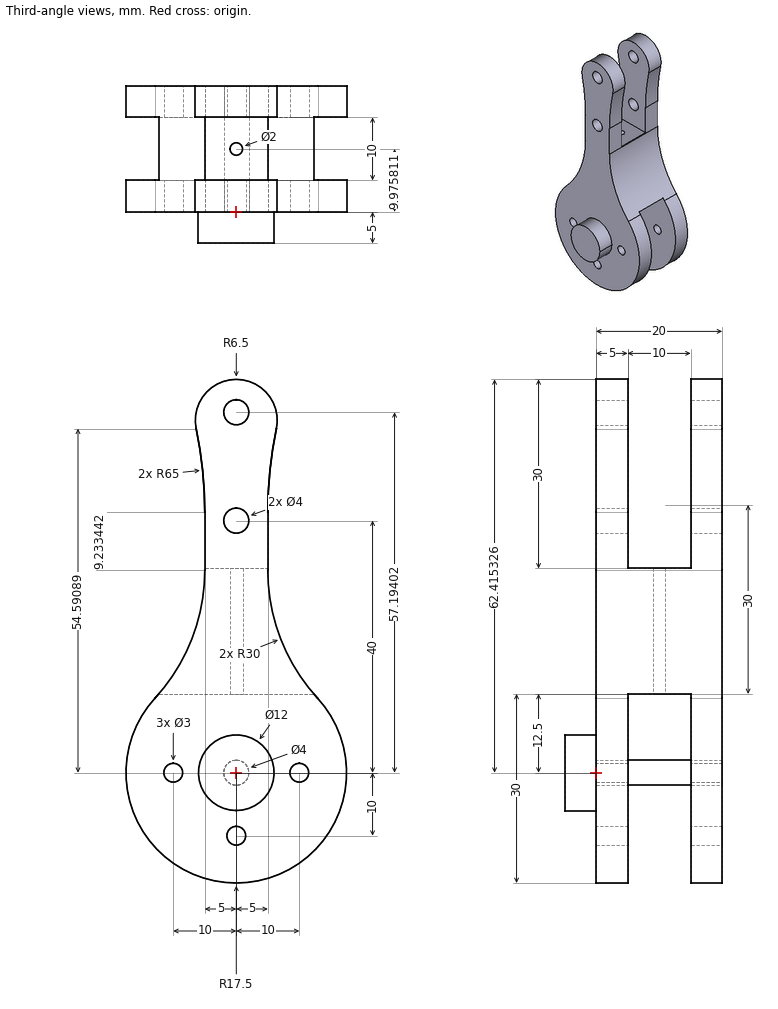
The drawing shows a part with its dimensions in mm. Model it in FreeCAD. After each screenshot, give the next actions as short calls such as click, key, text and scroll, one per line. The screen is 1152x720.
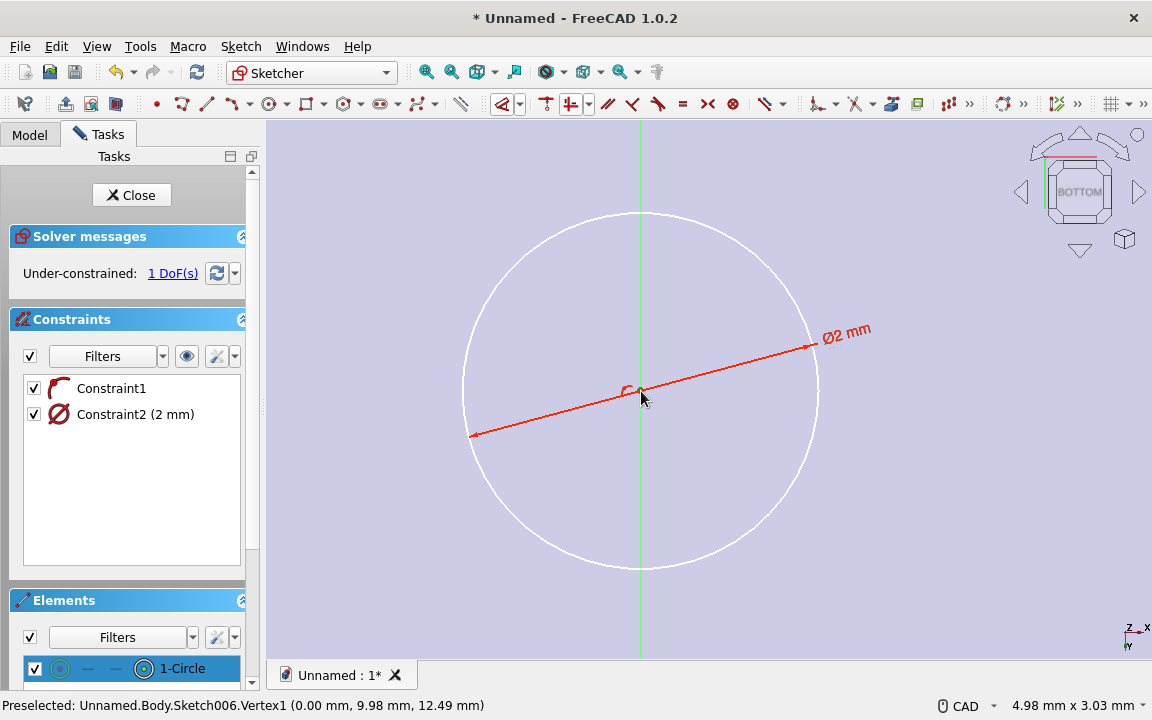
key(i)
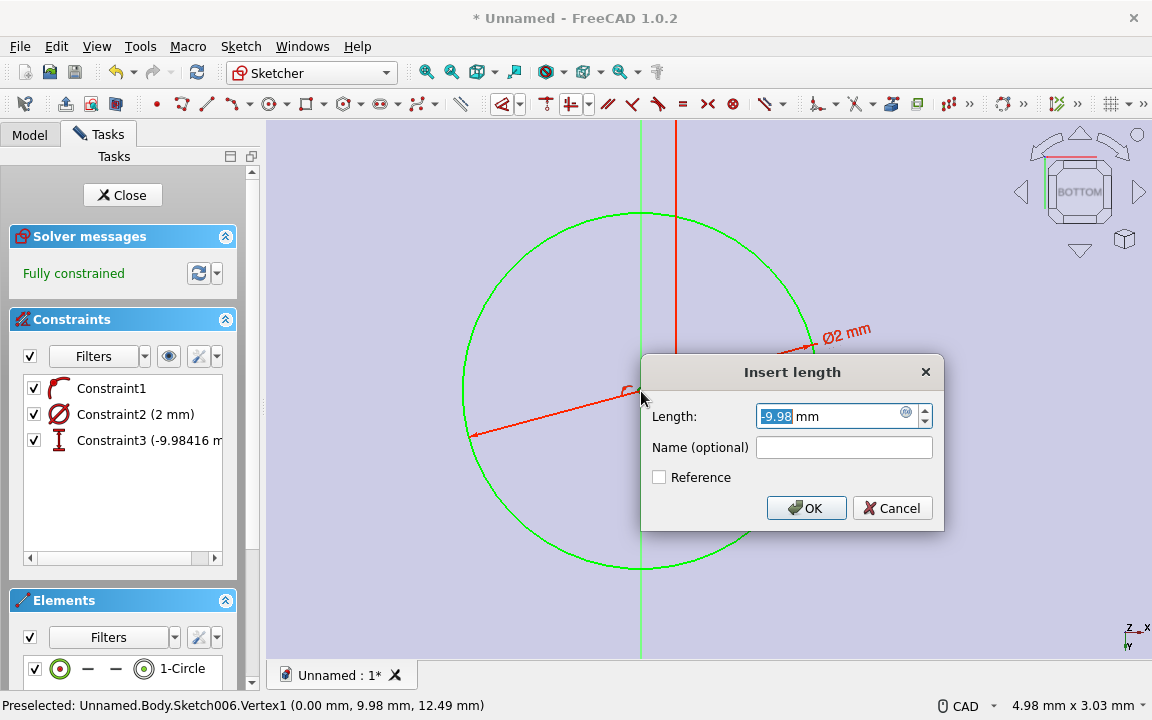
text(-9.975811)
key(Return)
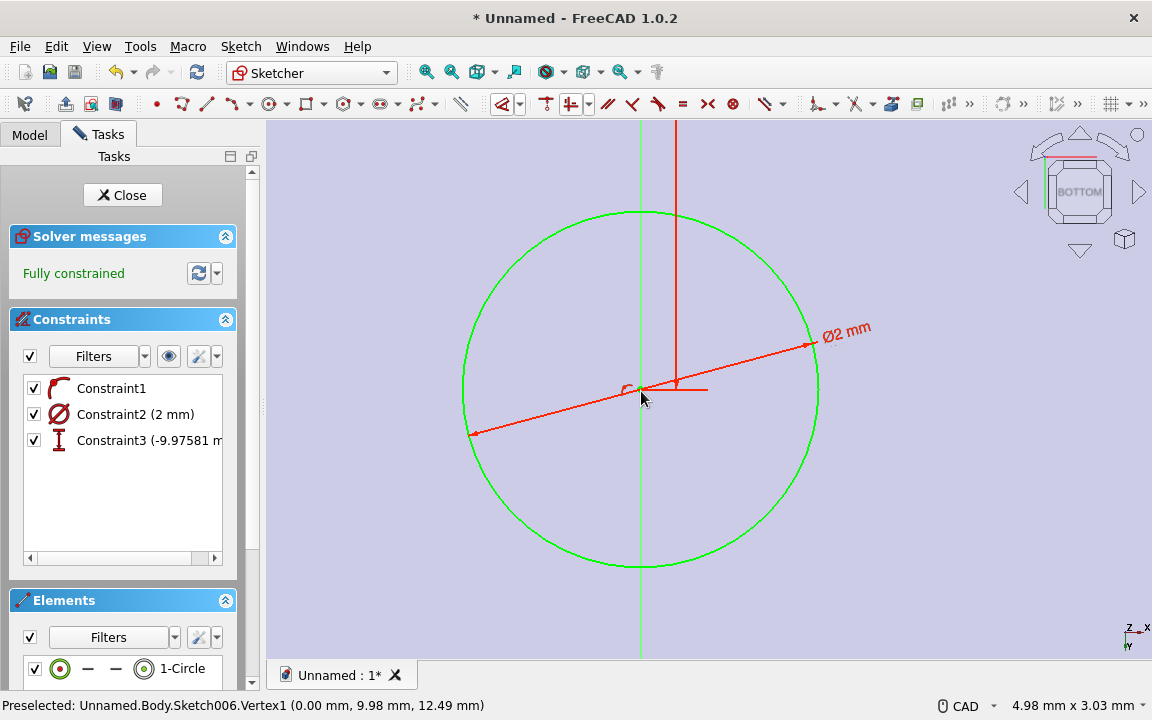
click(123, 195)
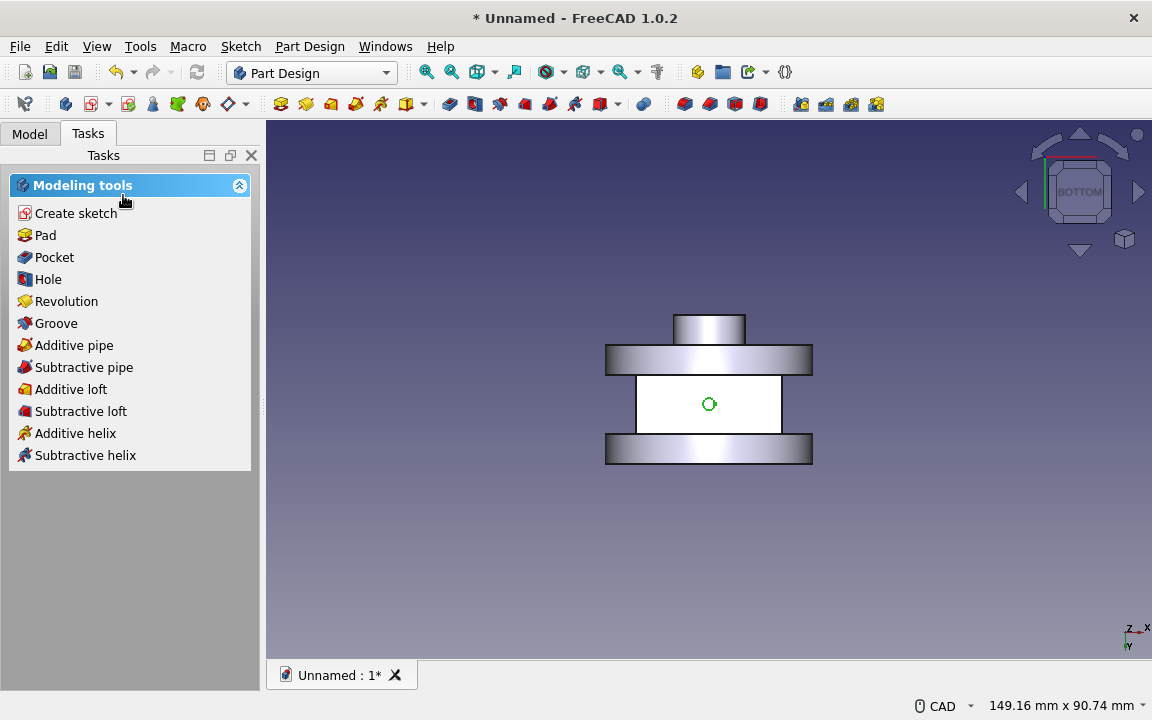
click(450, 104)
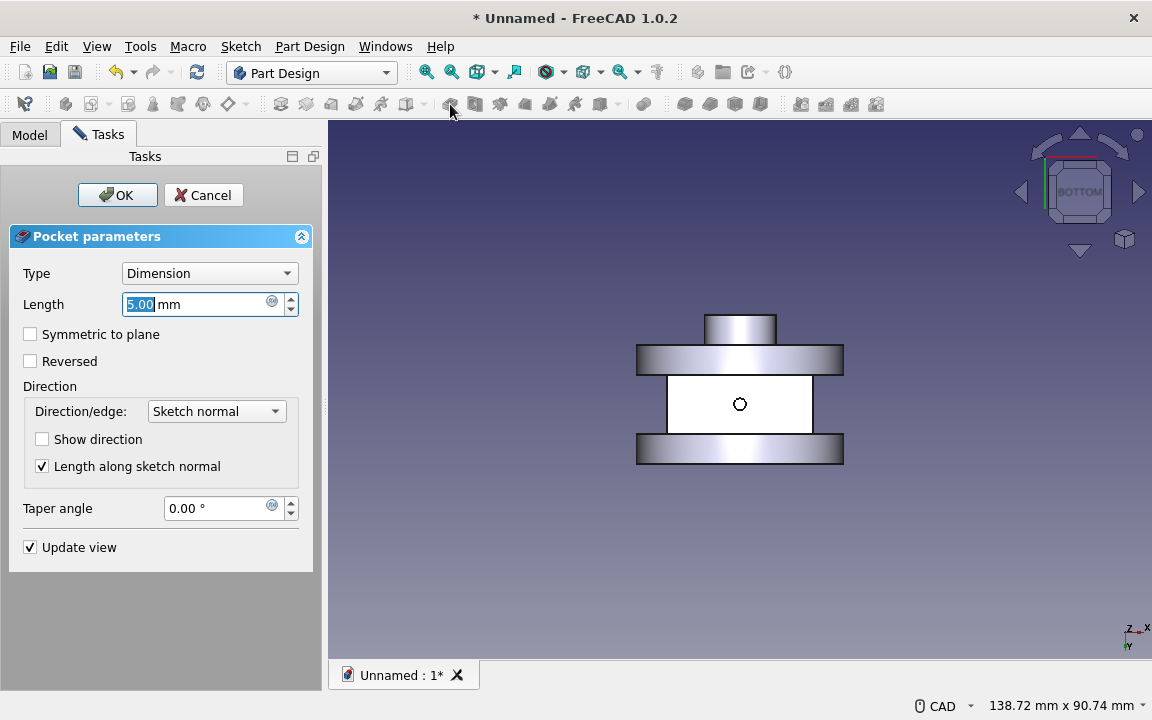
text(30)
key(Tab)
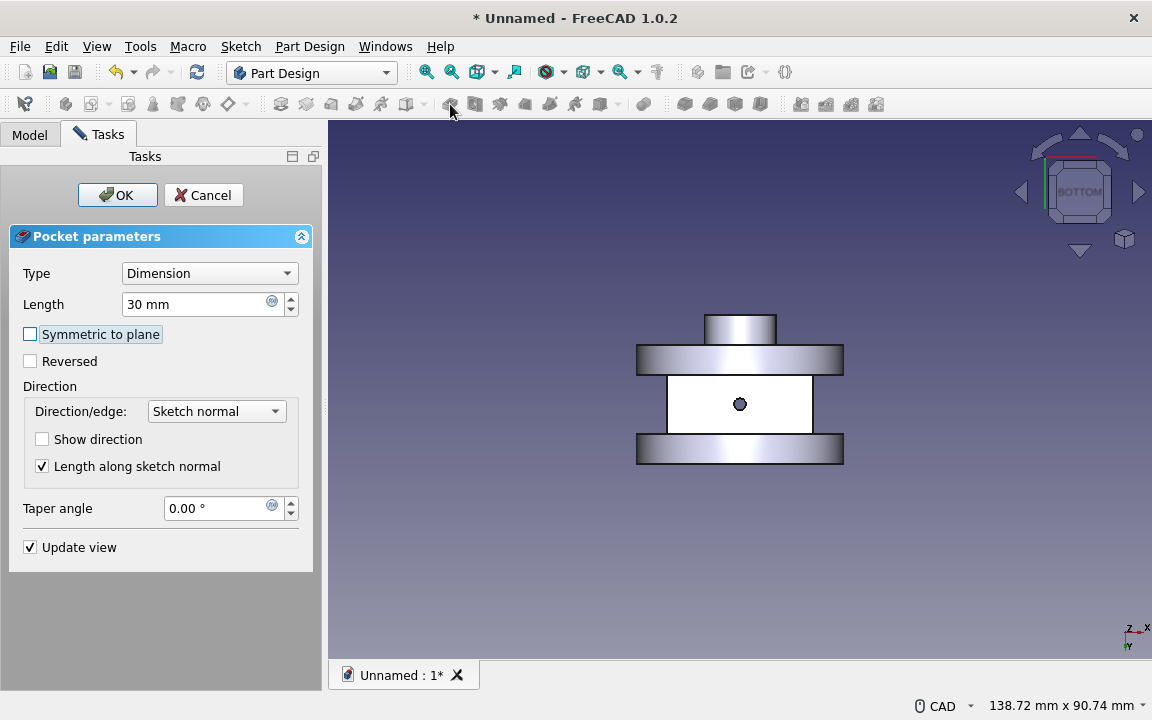
click(118, 195)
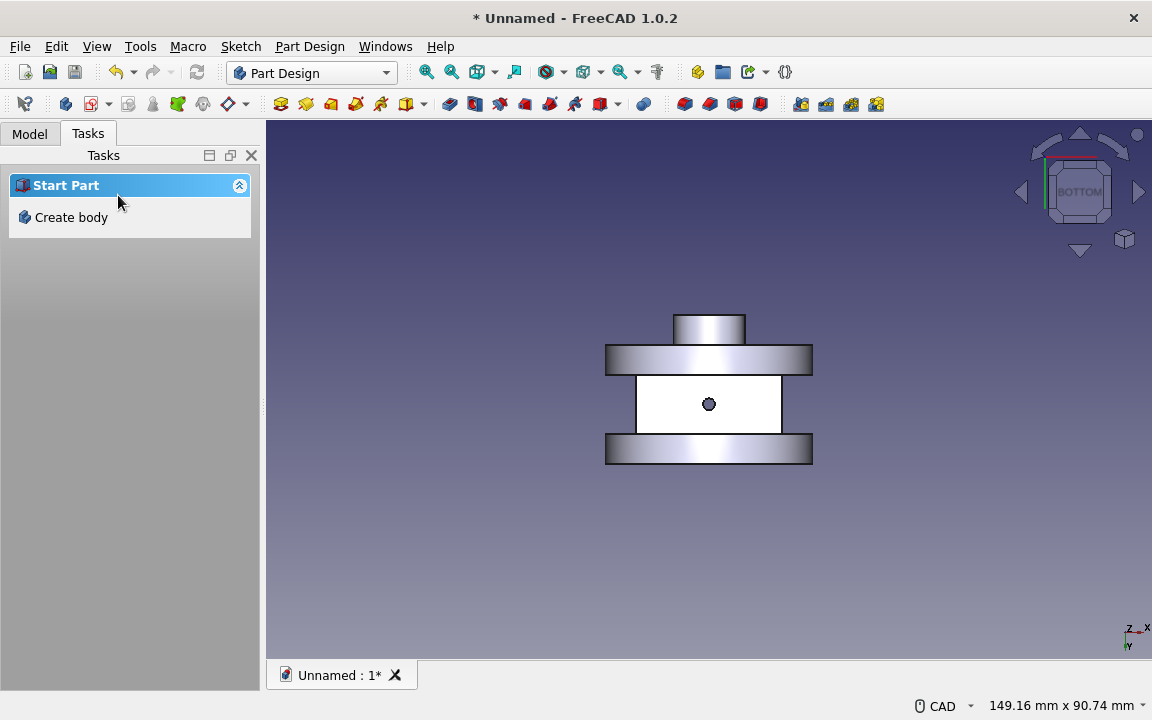
click(427, 72)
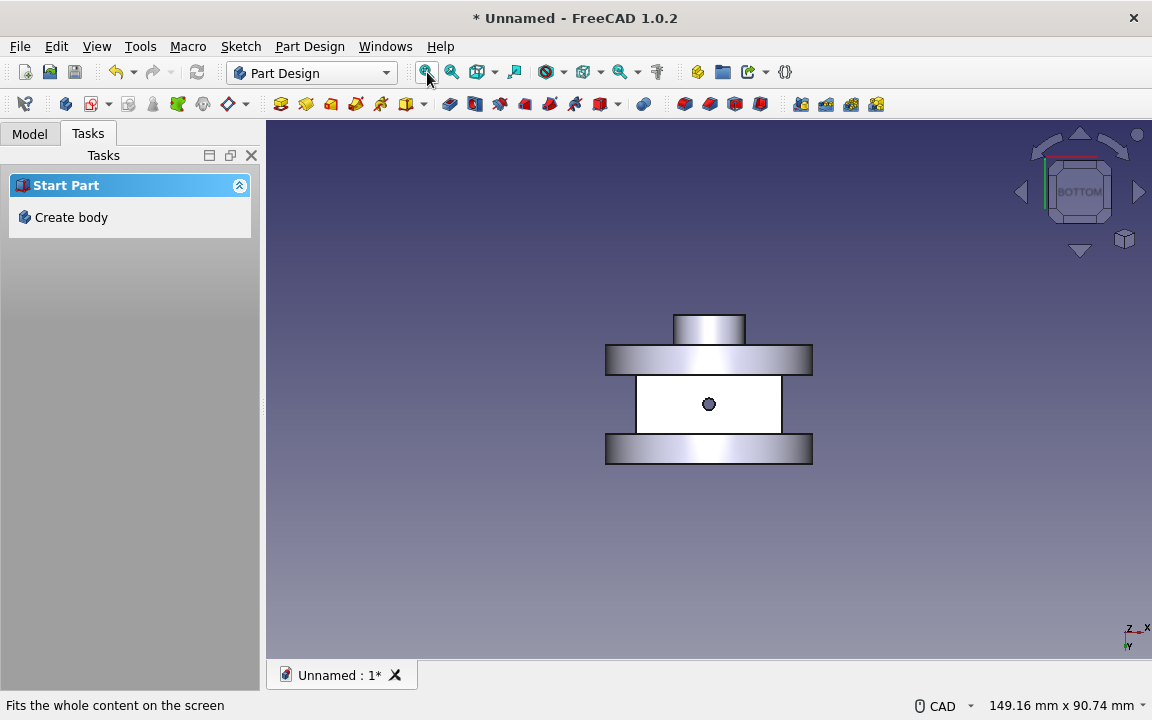
click(66, 104)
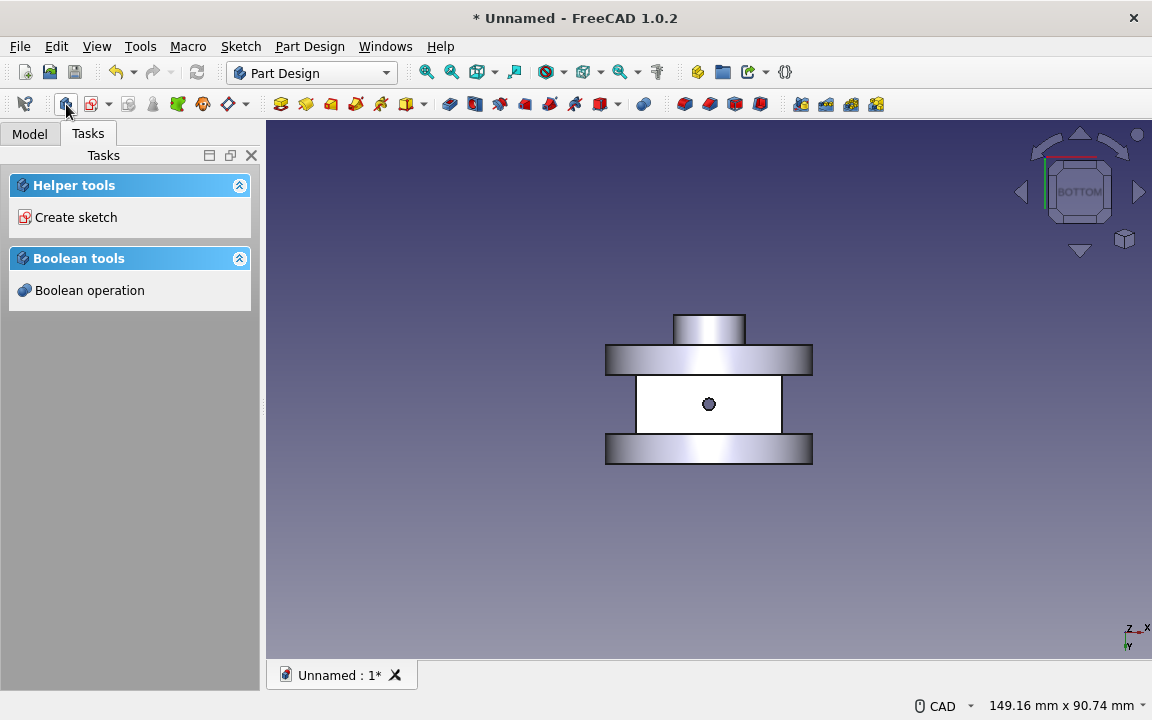
click(30, 134)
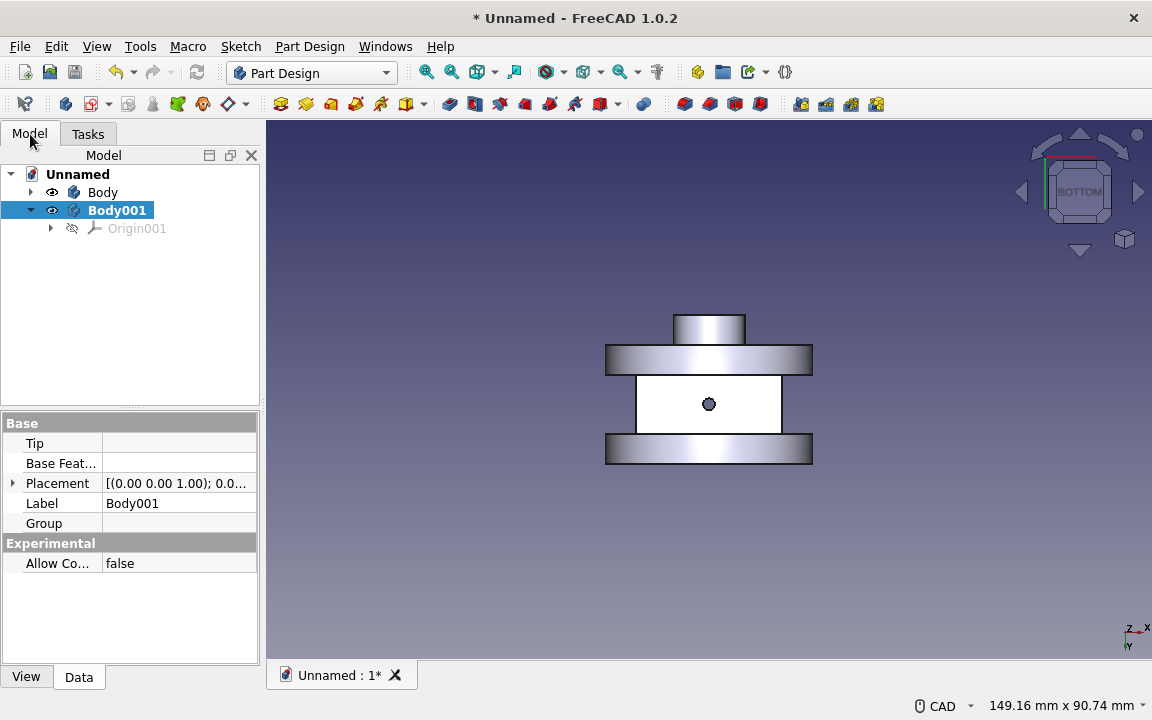
click(51, 228)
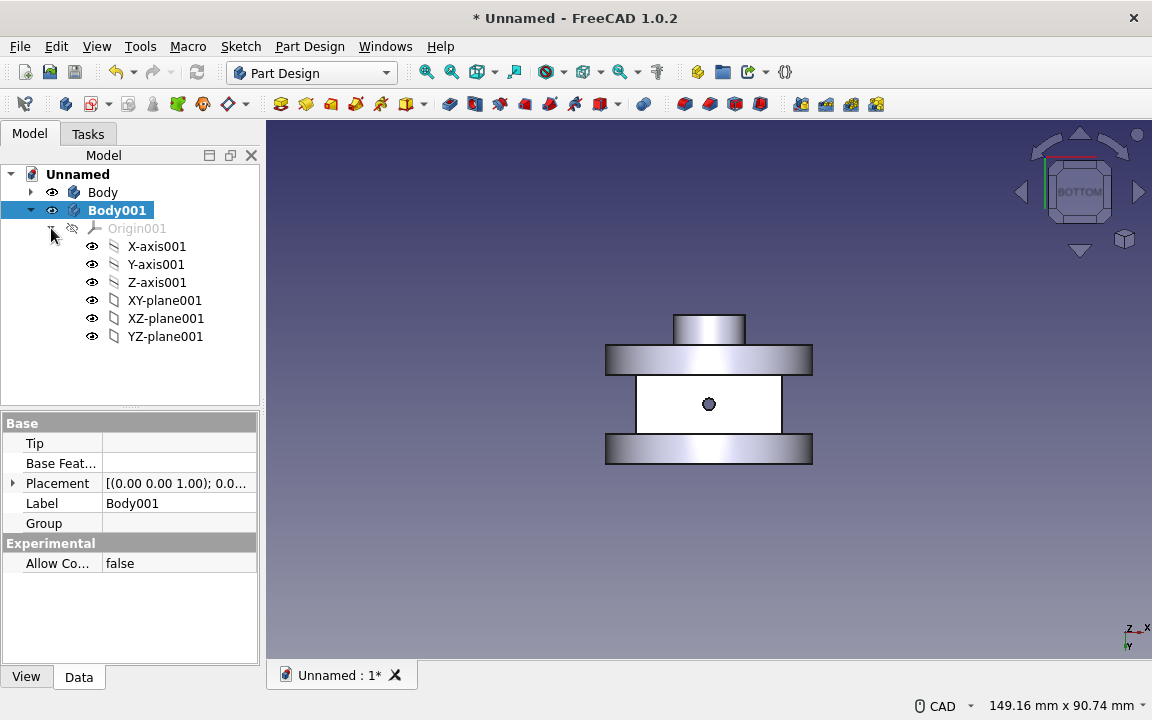
click(137, 318)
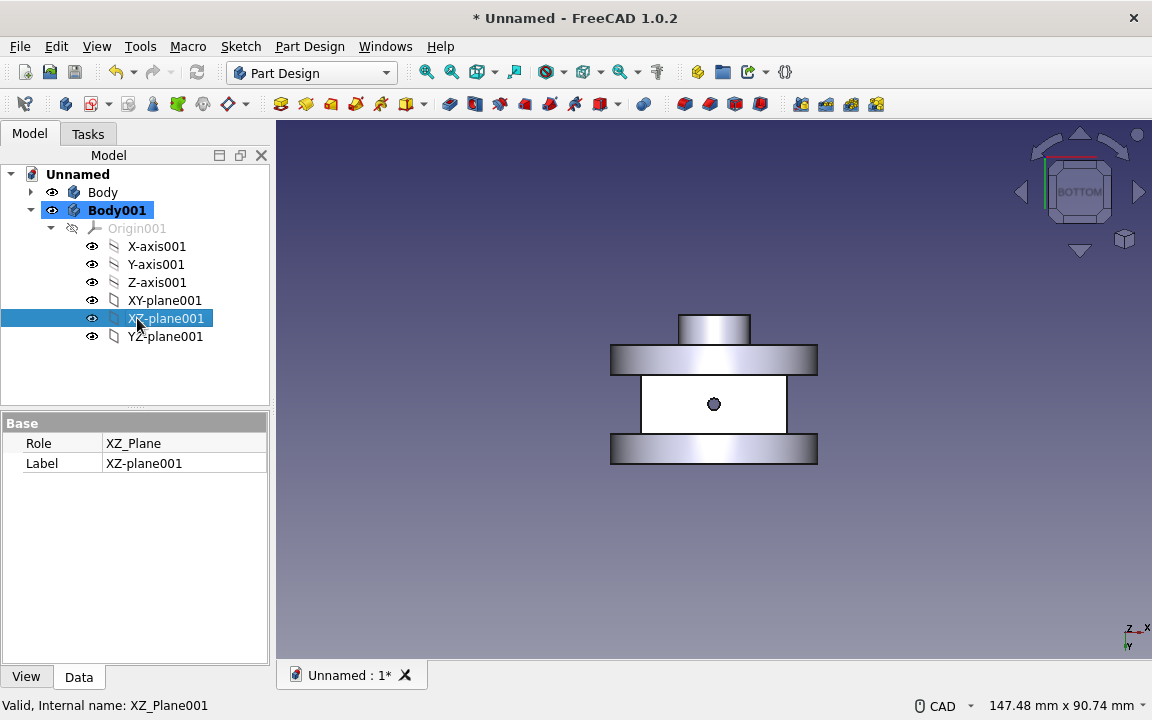
click(228, 104)